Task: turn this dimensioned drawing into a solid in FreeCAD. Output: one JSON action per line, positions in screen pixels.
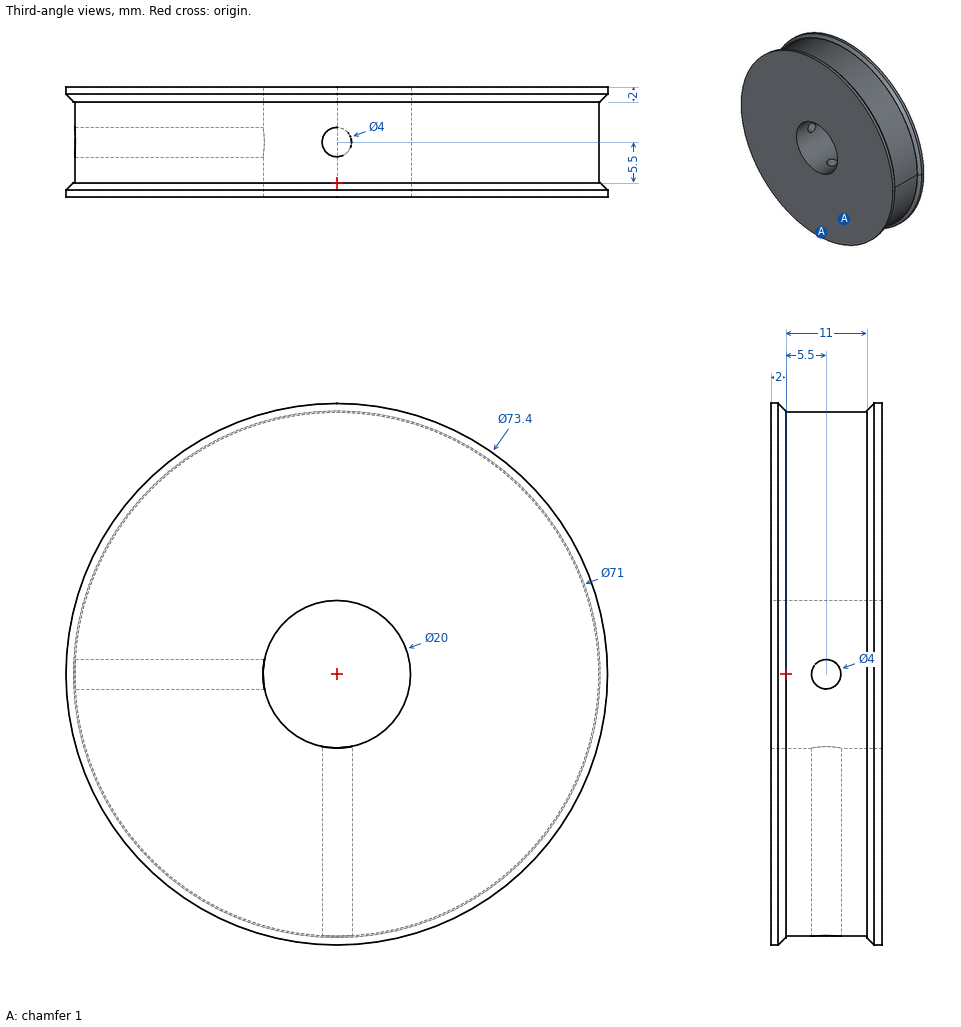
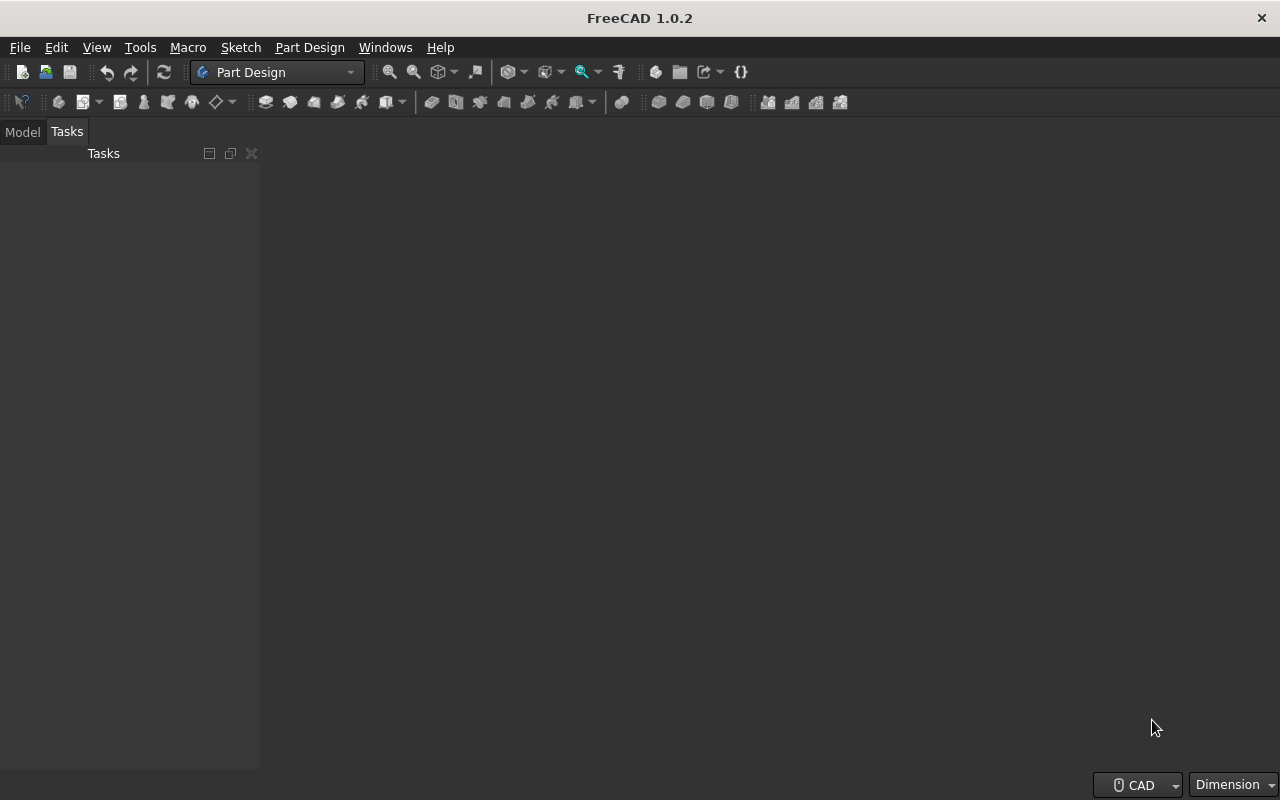
{"action": "left_click", "coordinate": [22, 72]}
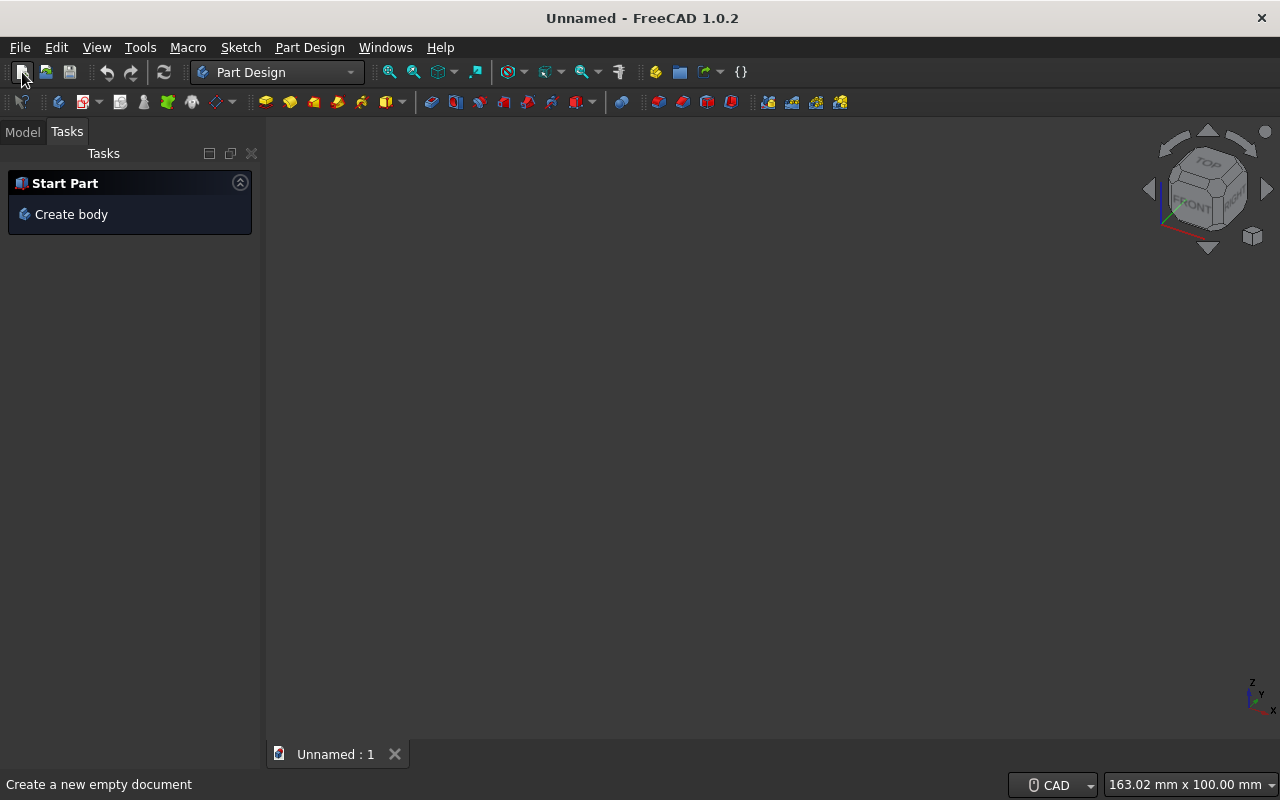
{"action": "left_click", "coordinate": [84, 102]}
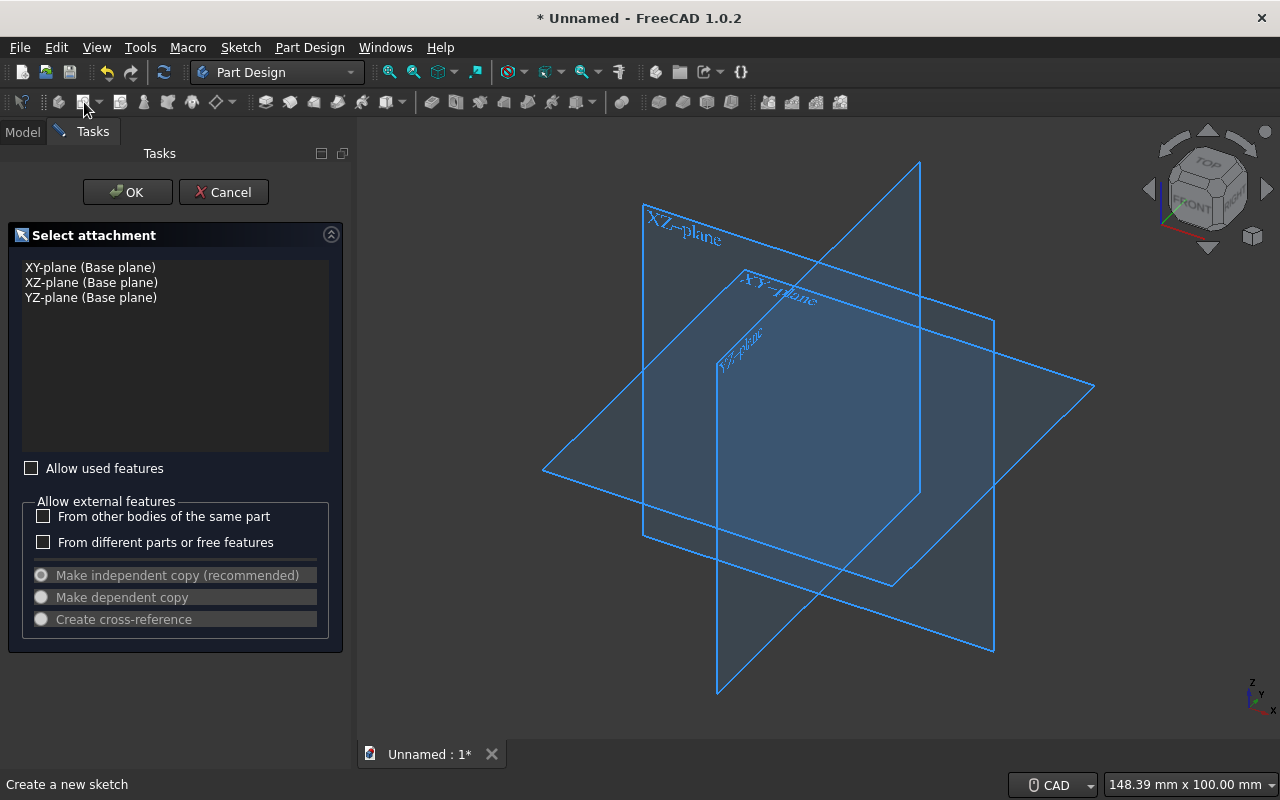
{"action": "left_click", "coordinate": [82, 282]}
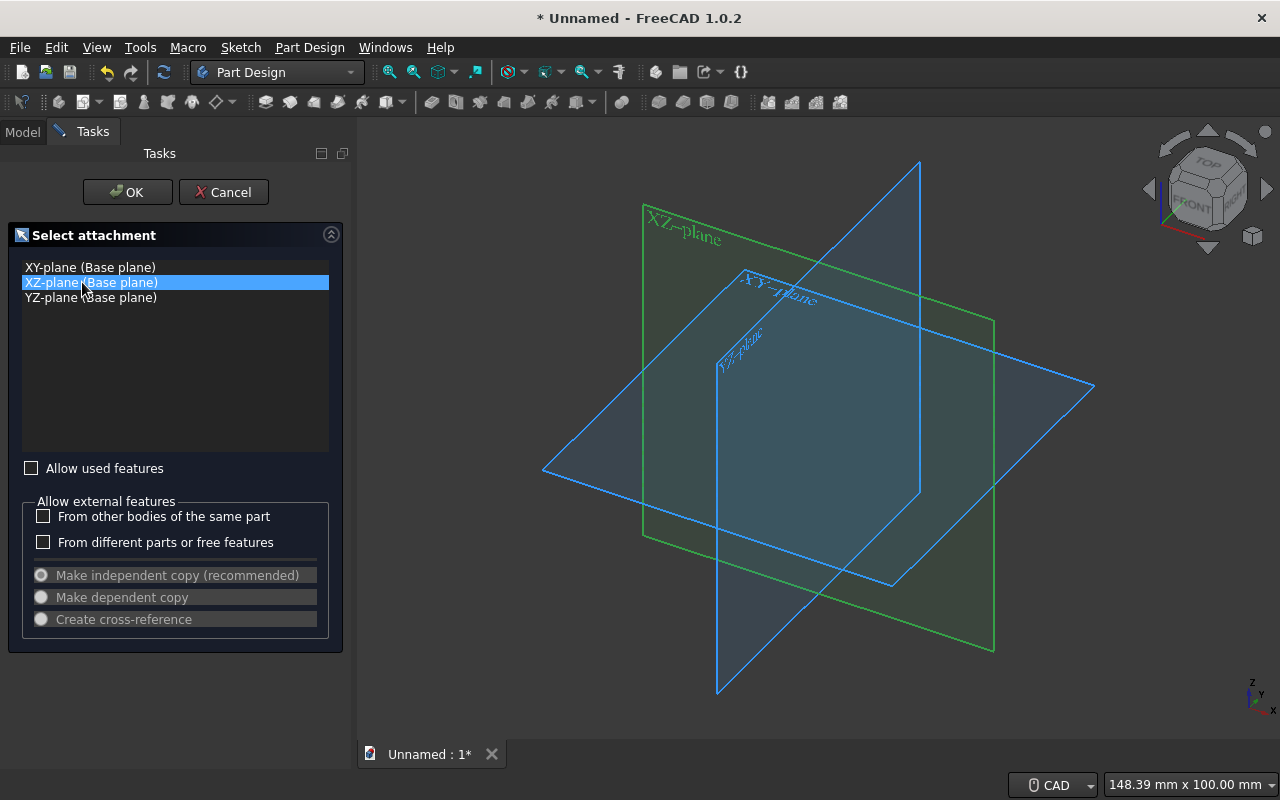
{"action": "left_click", "coordinate": [128, 192]}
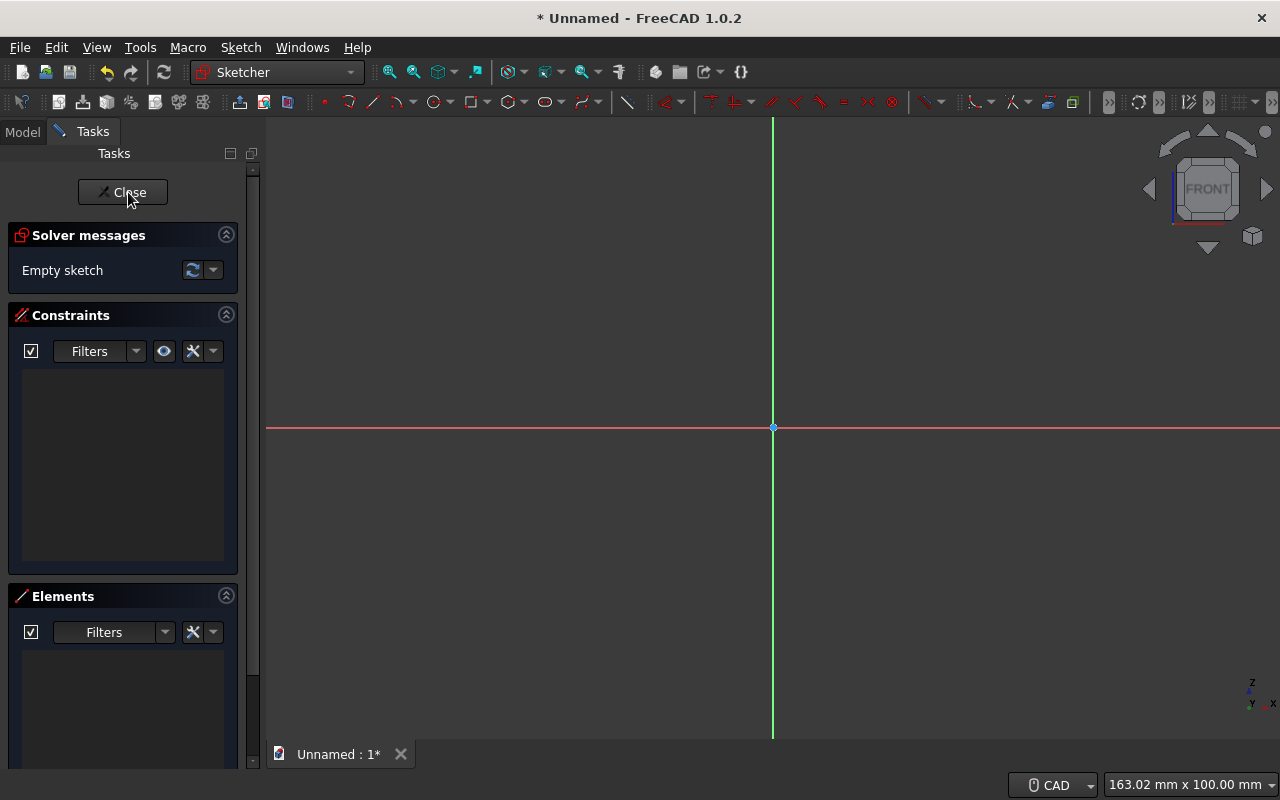
{"action": "left_click", "coordinate": [434, 102]}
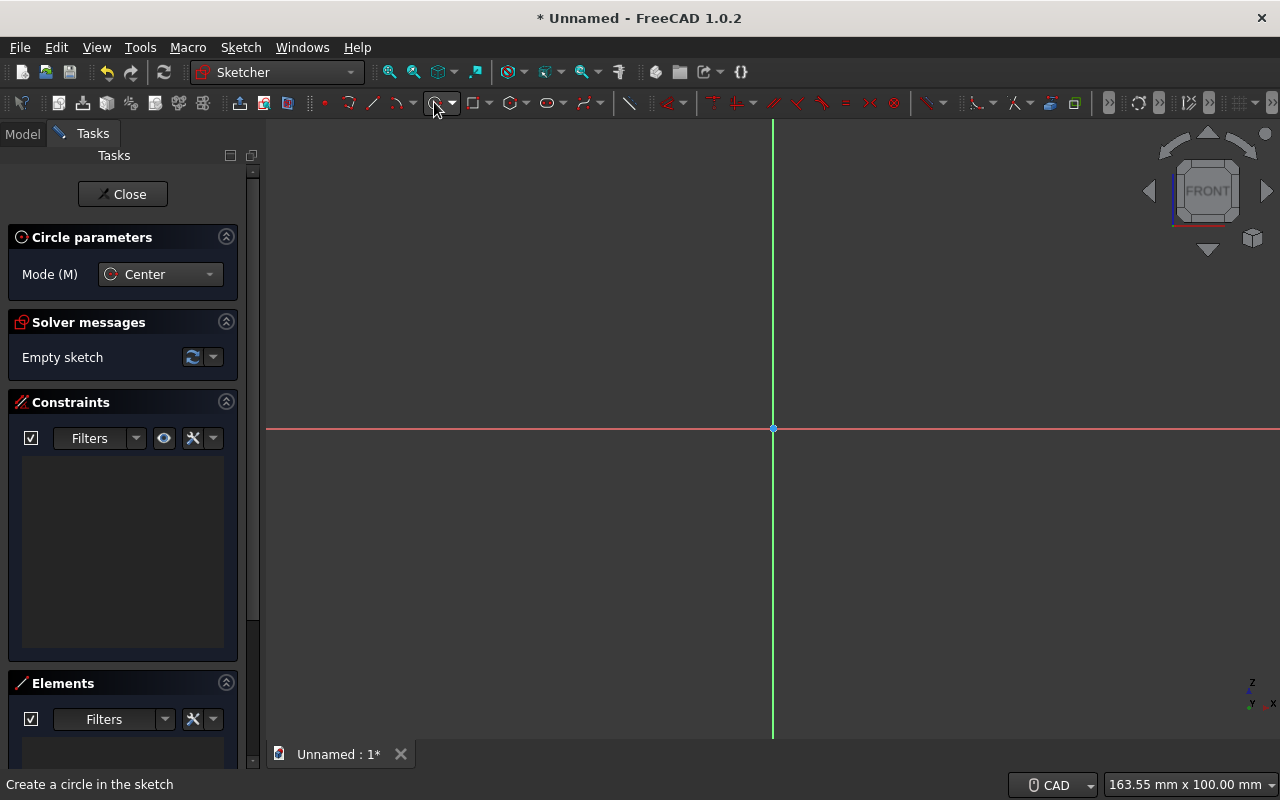
{"action": "left_click", "coordinate": [773, 429]}
{"action": "left_click", "coordinate": [929, 273]}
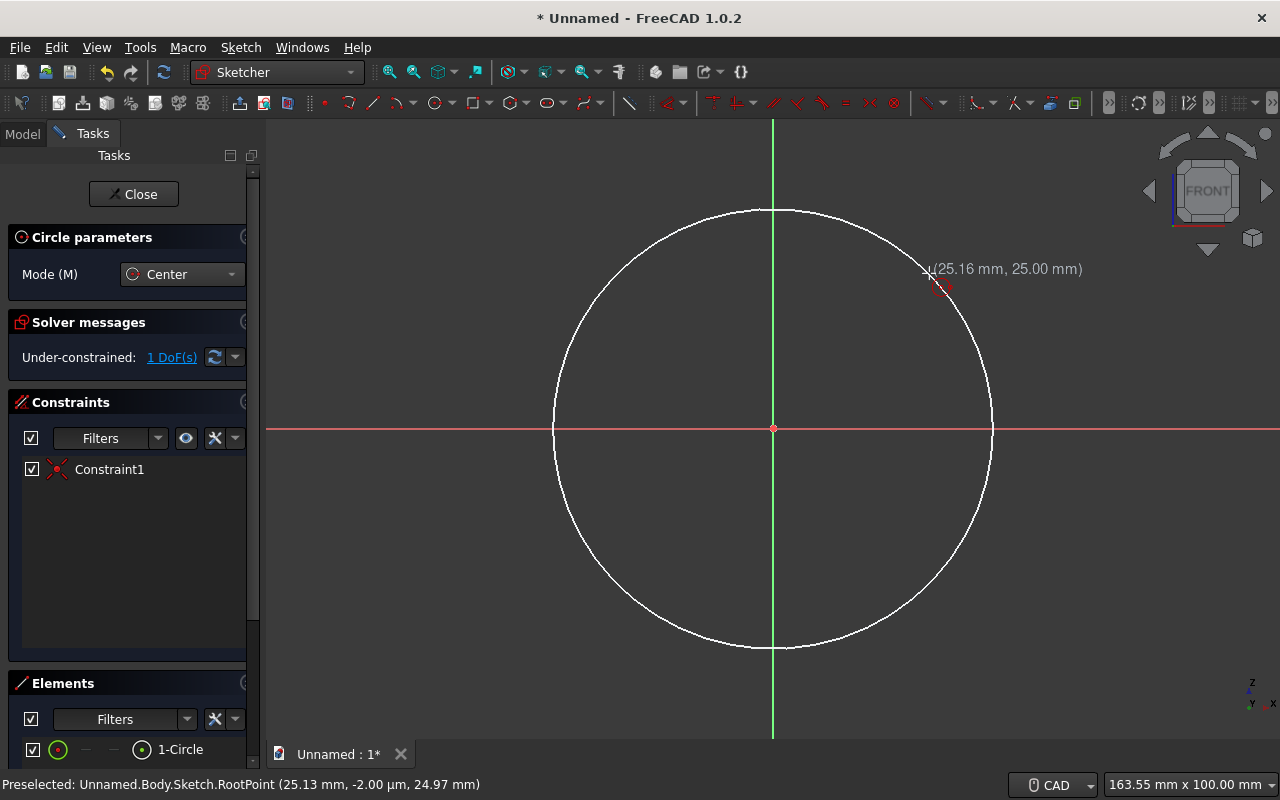
{"action": "left_click", "coordinate": [773, 429]}
{"action": "left_click", "coordinate": [817, 385]}
{"action": "key", "text": "Escape"}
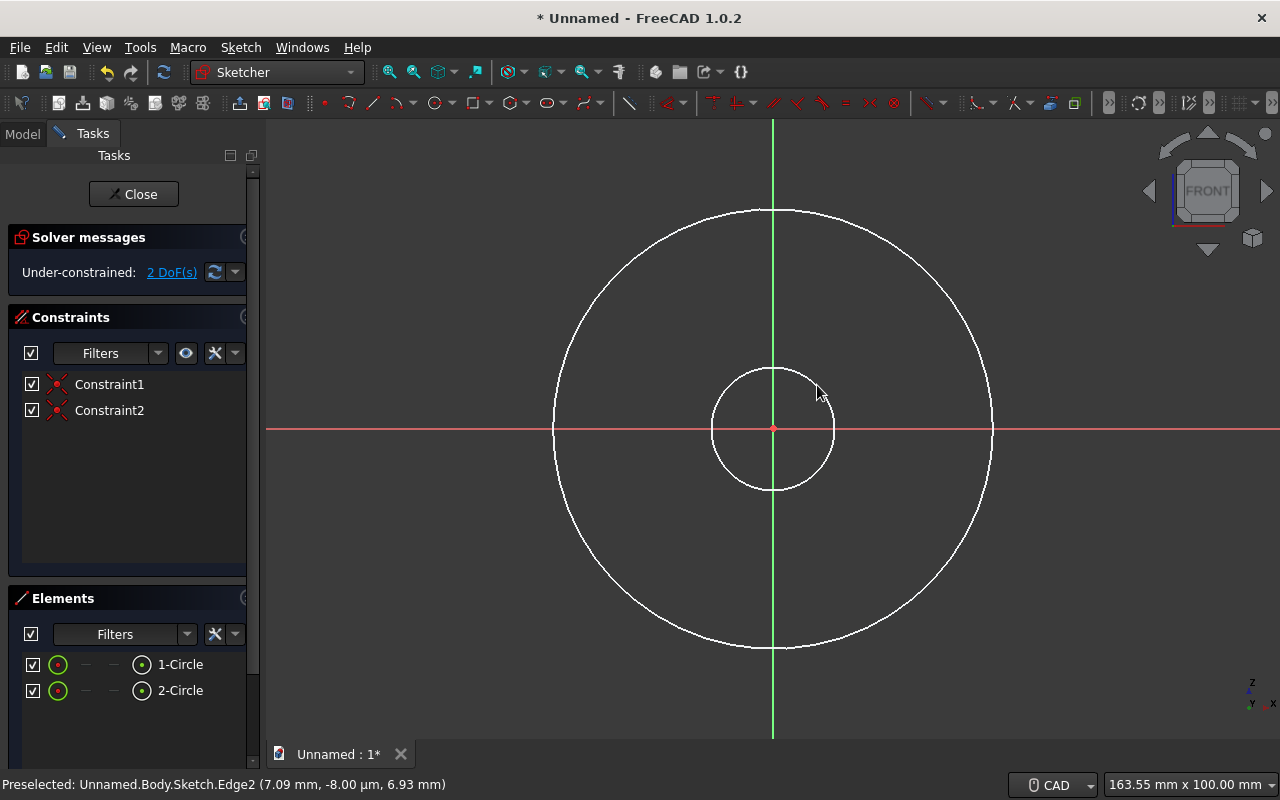
{"action": "left_click", "coordinate": [668, 104]}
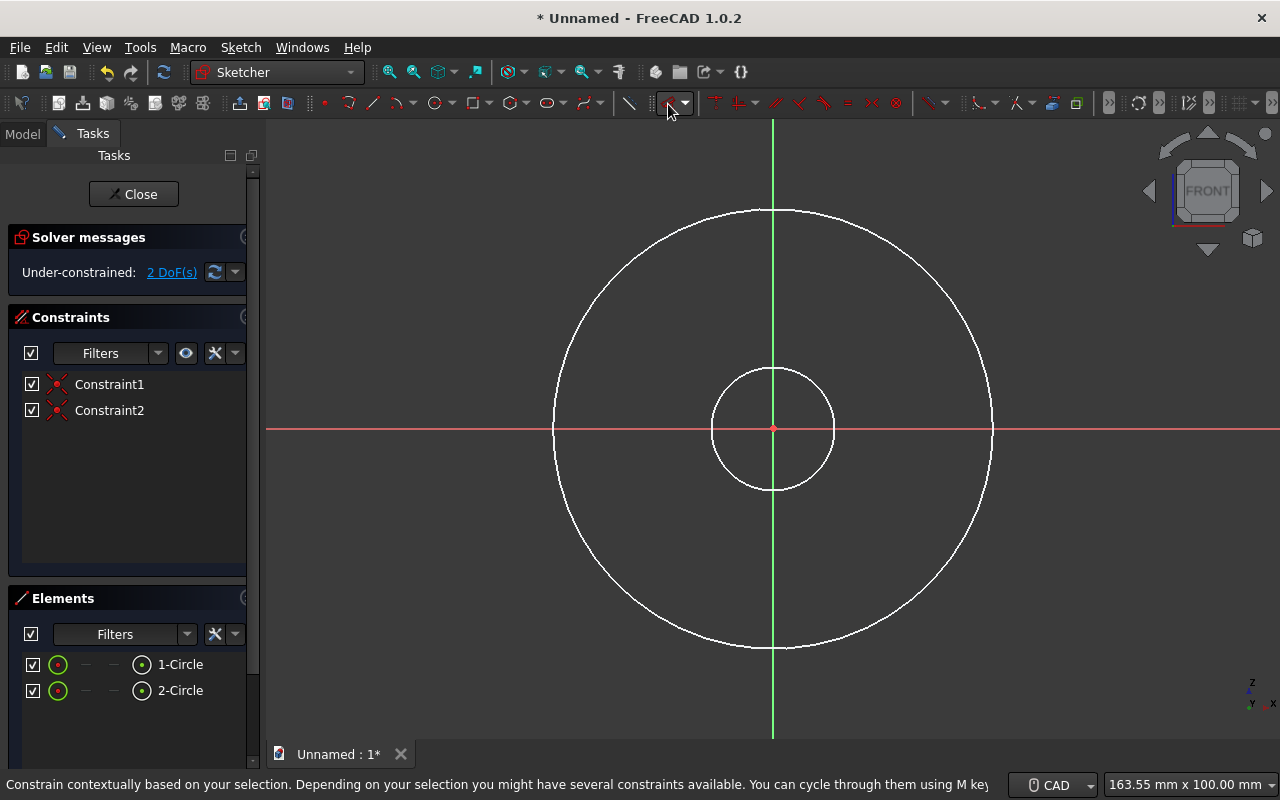
{"action": "left_click", "coordinate": [928, 273]}
{"action": "left_click", "coordinate": [951, 250]}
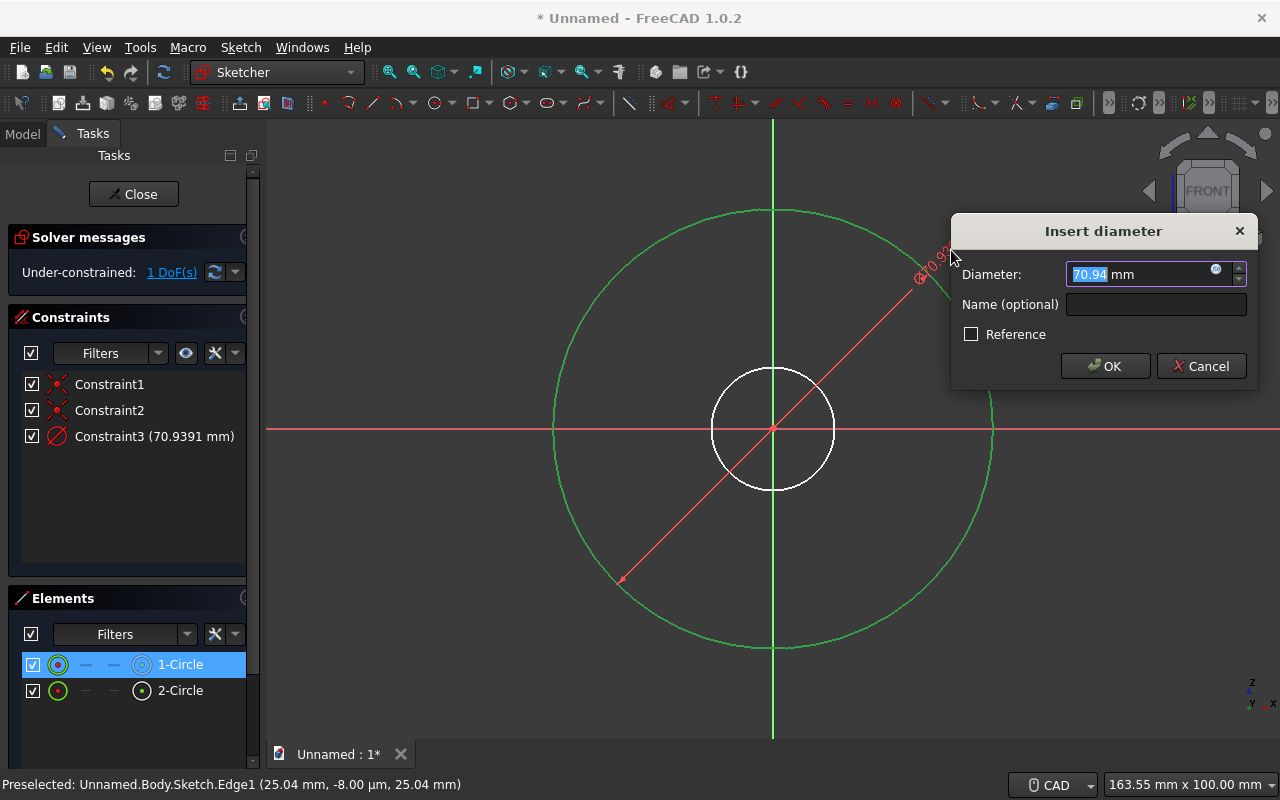
{"action": "type", "text": "71"}
{"action": "key", "text": "Return"}